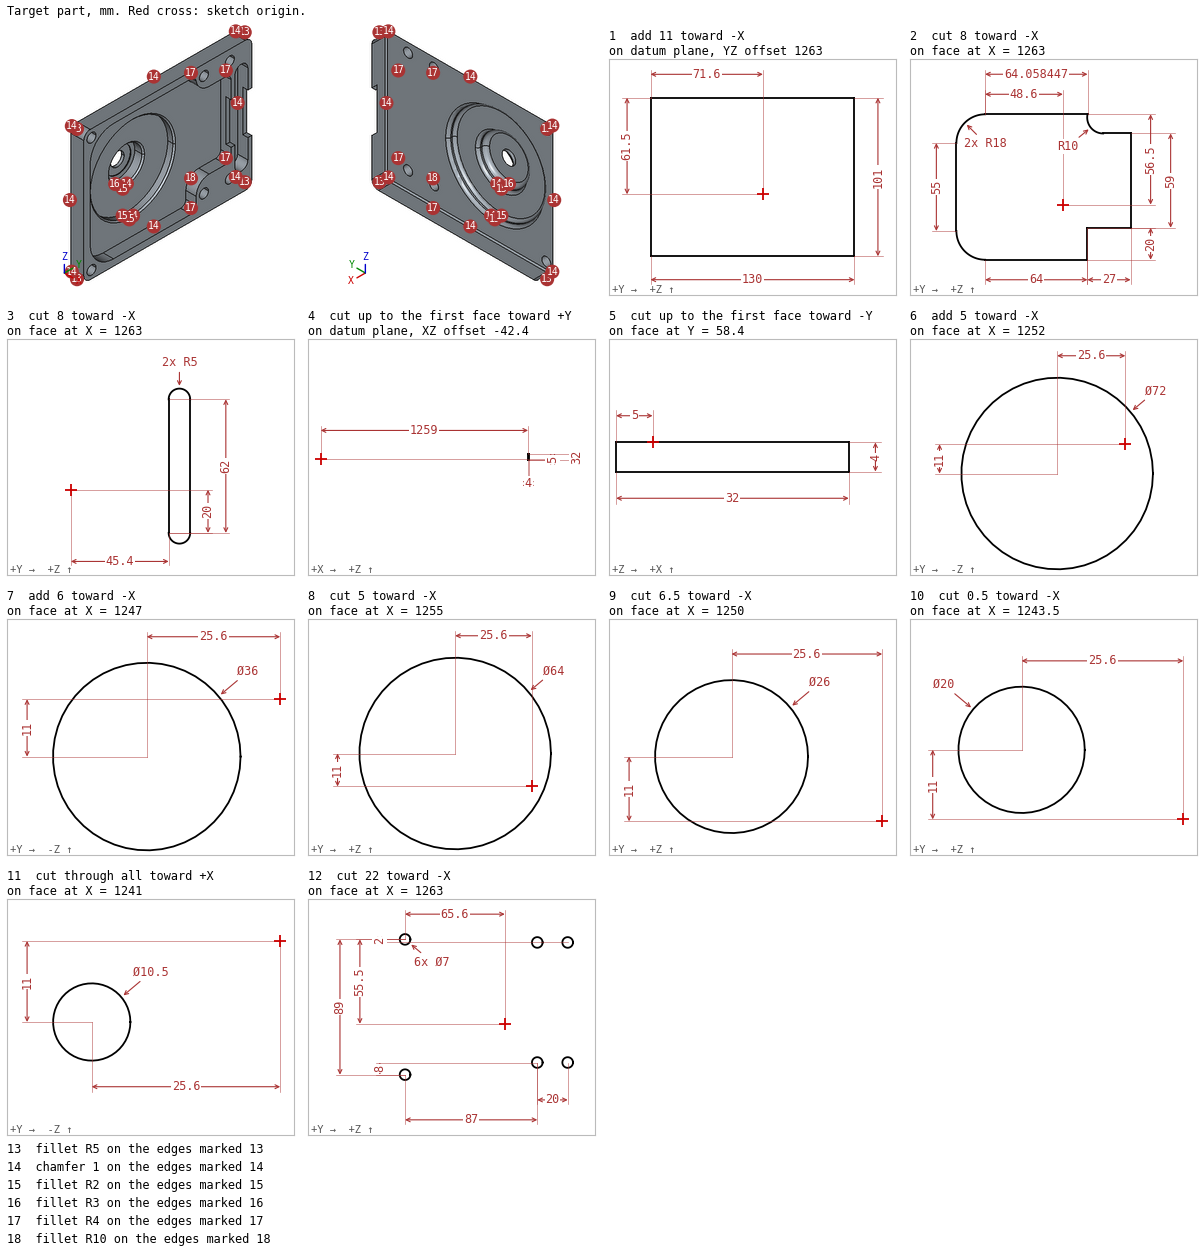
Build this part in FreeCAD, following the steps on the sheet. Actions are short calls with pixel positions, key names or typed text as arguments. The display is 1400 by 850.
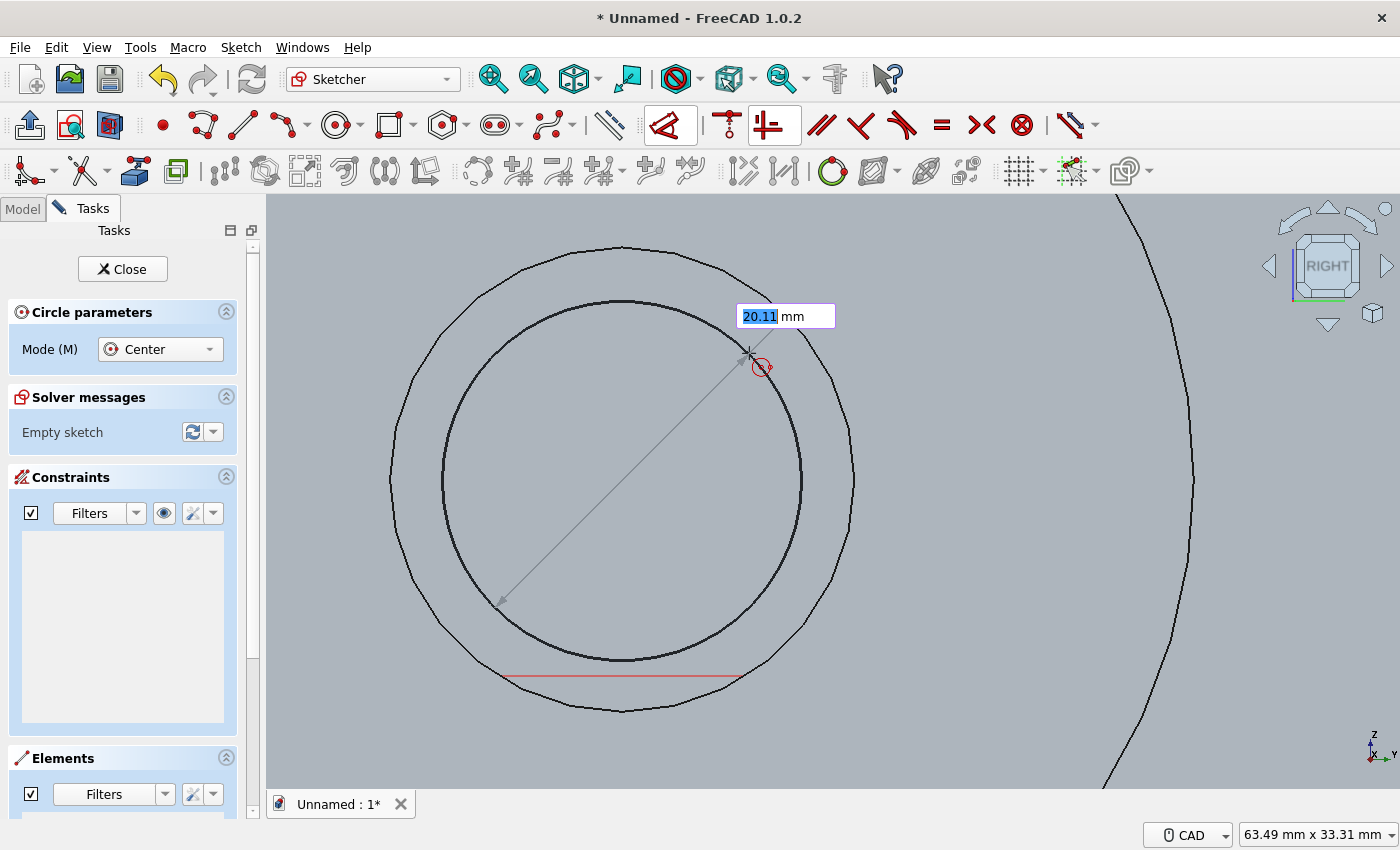
text(20)
key(Return)
key(Escape)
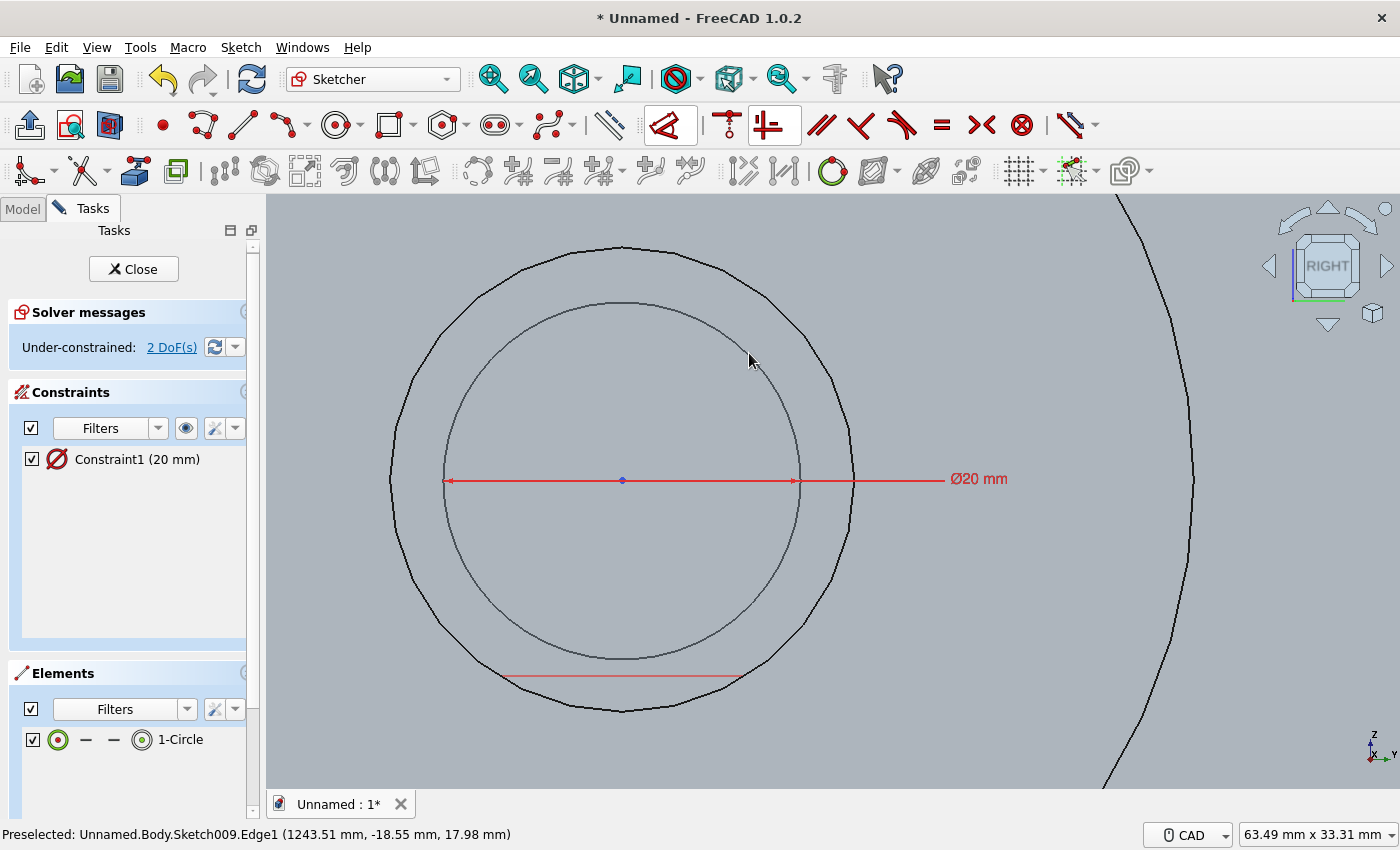
click(622, 481)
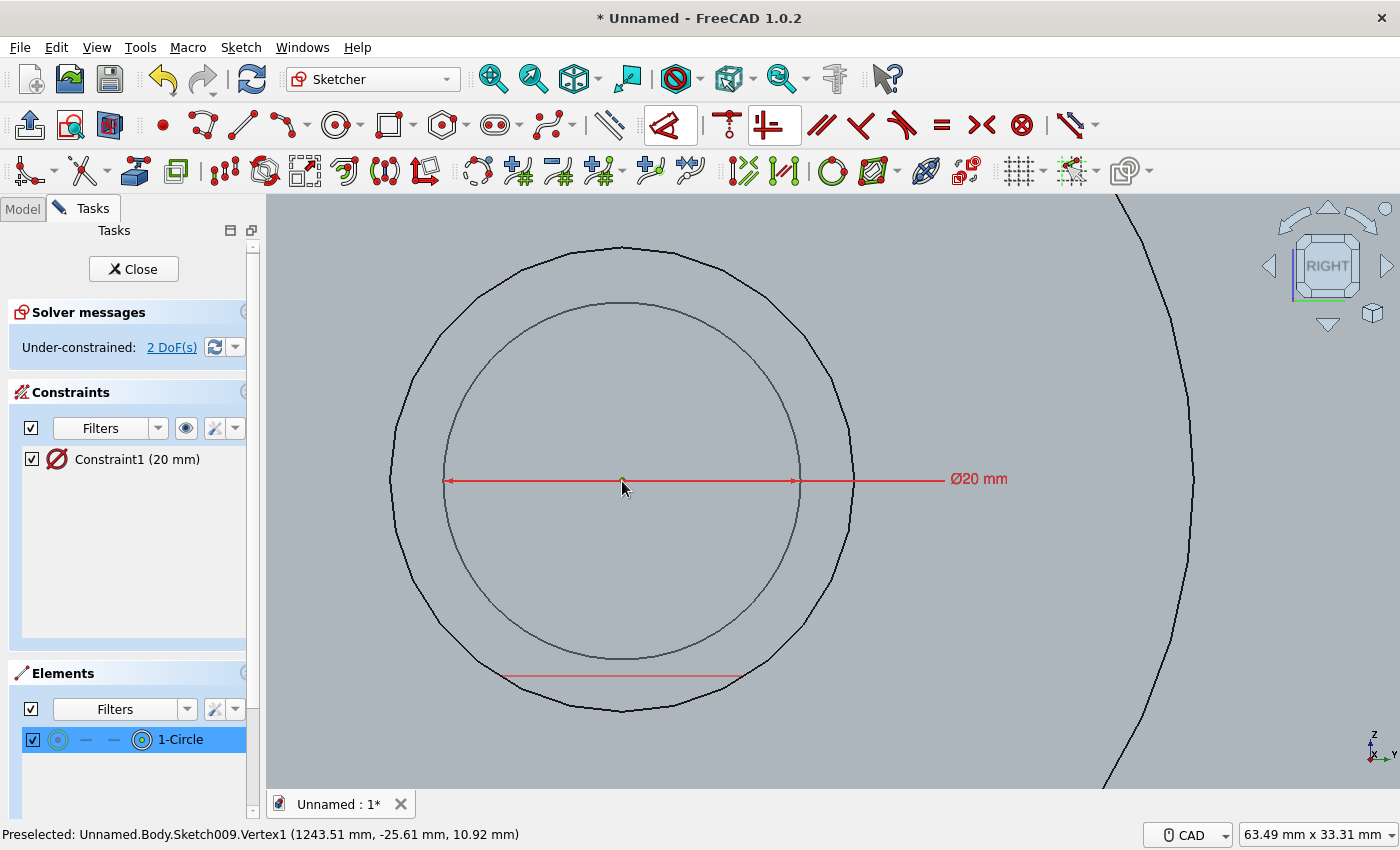
key(i)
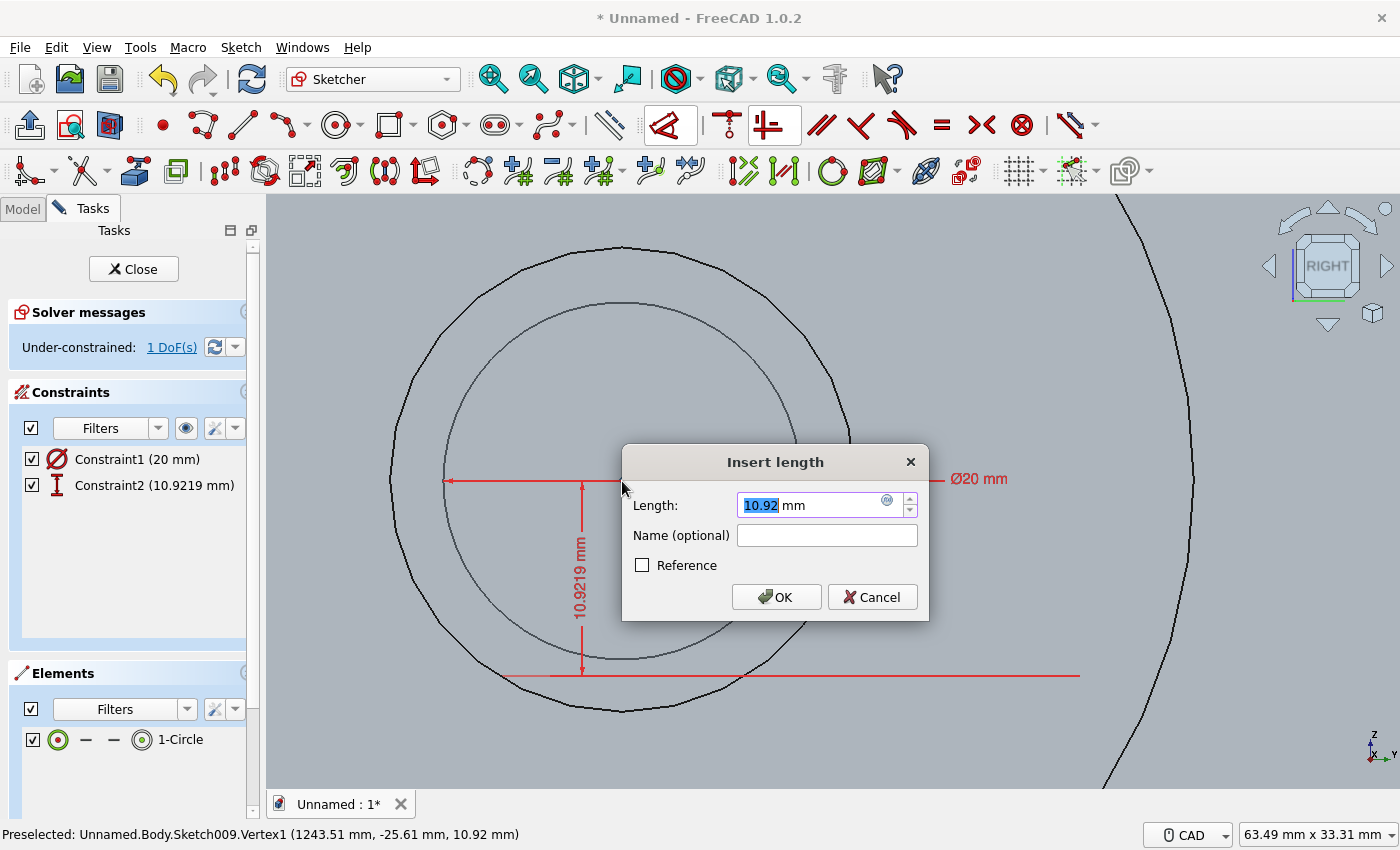
text(11)
key(Return)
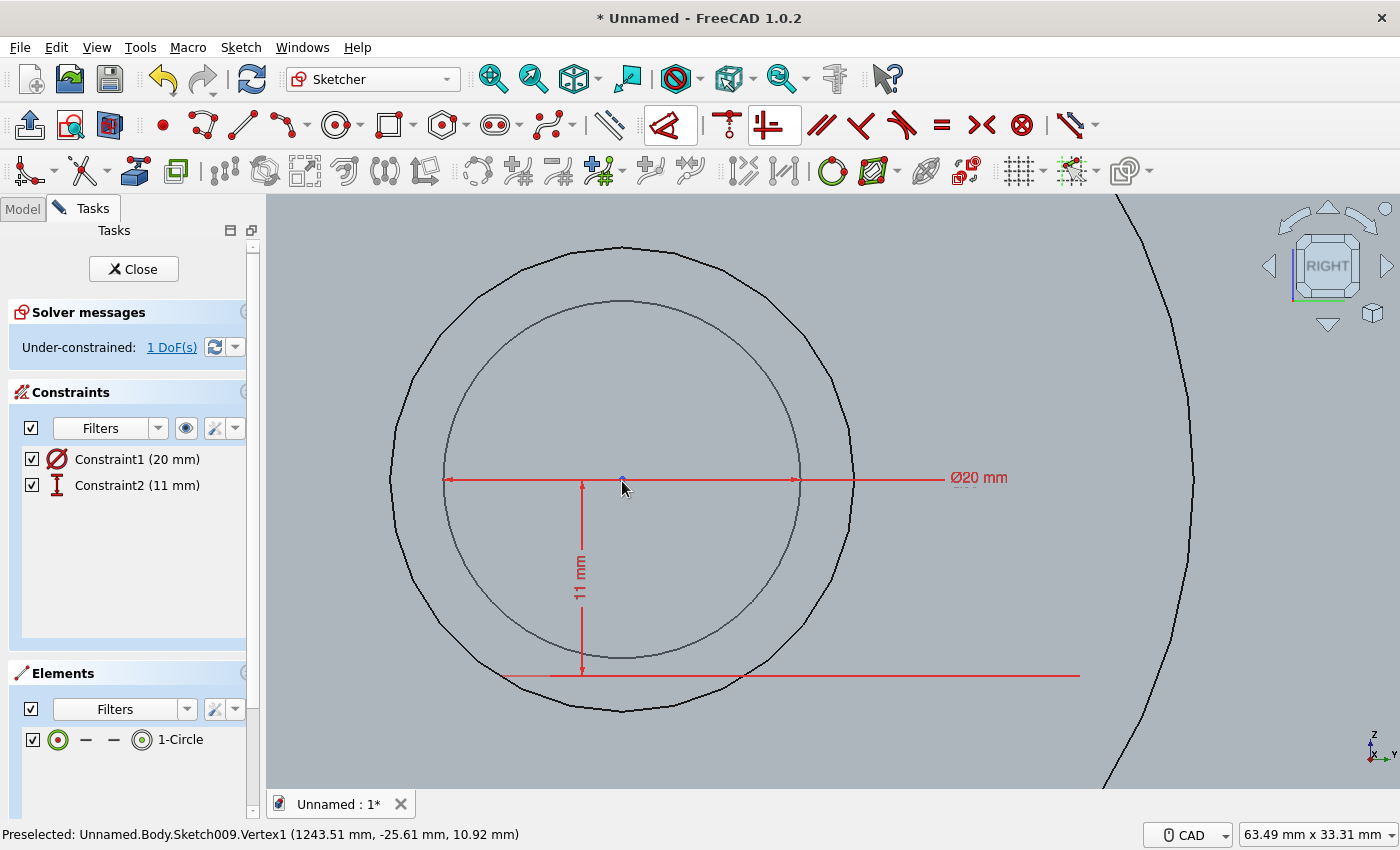
click(622, 480)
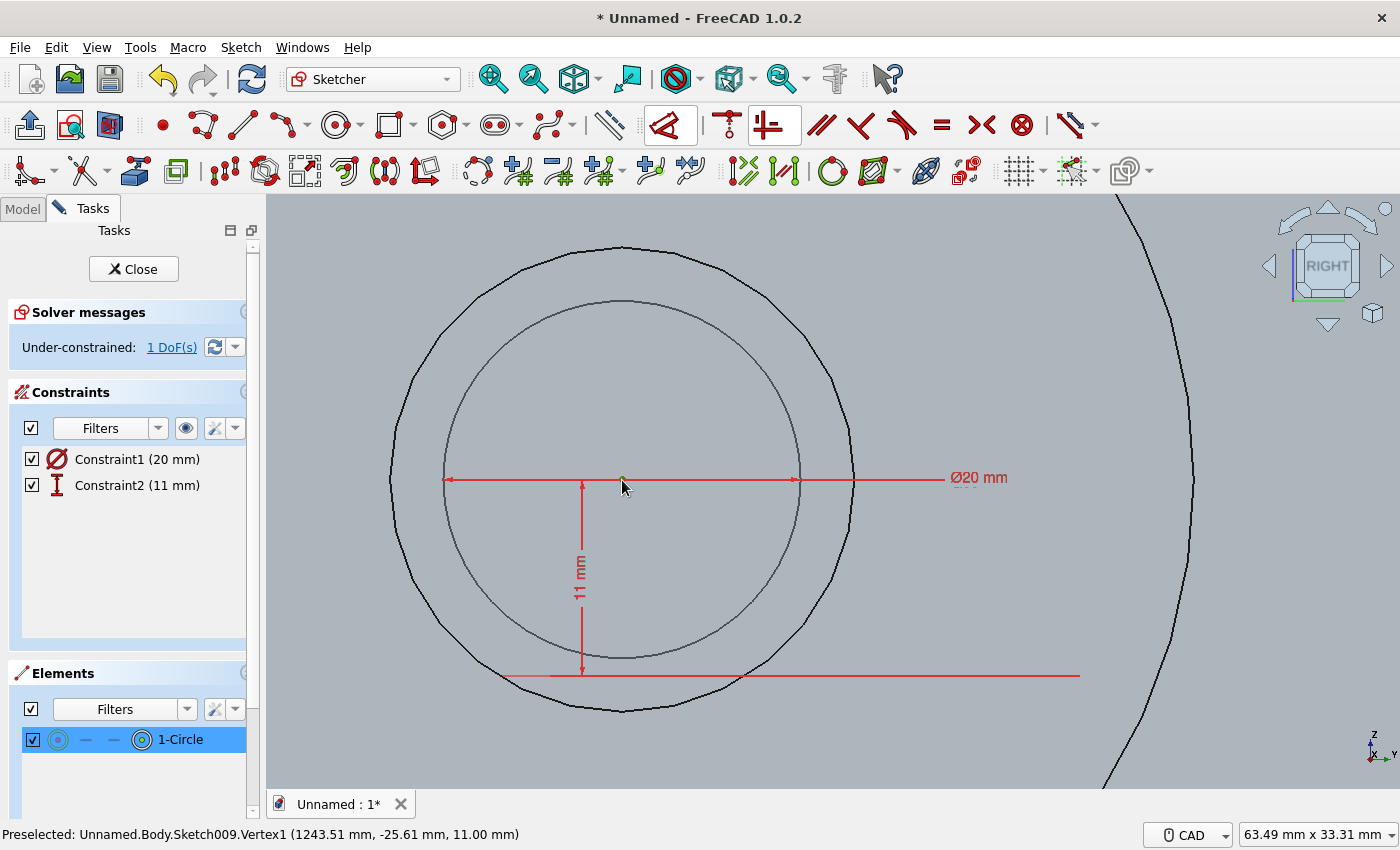
key(l)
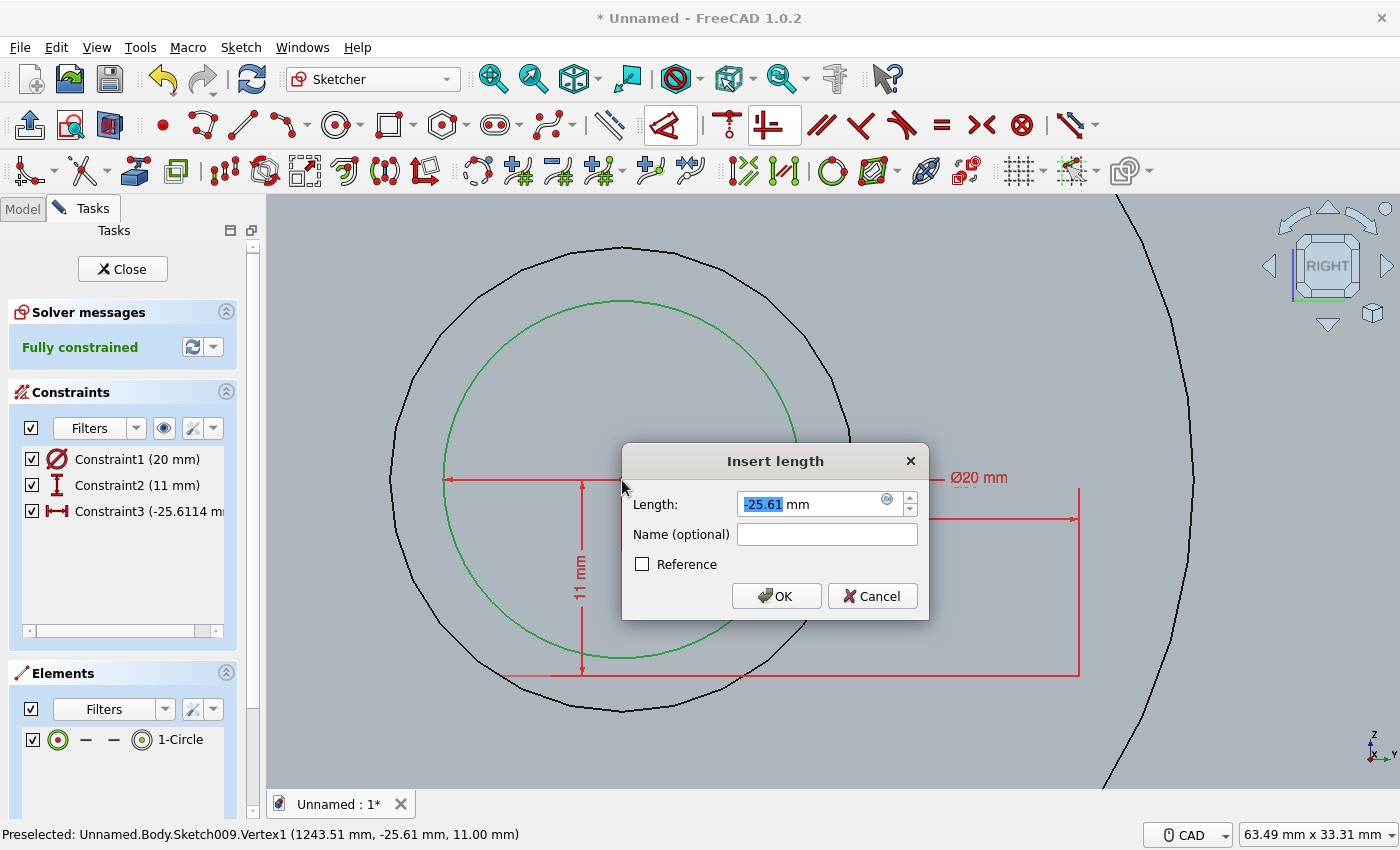
text(-25.6)
key(Return)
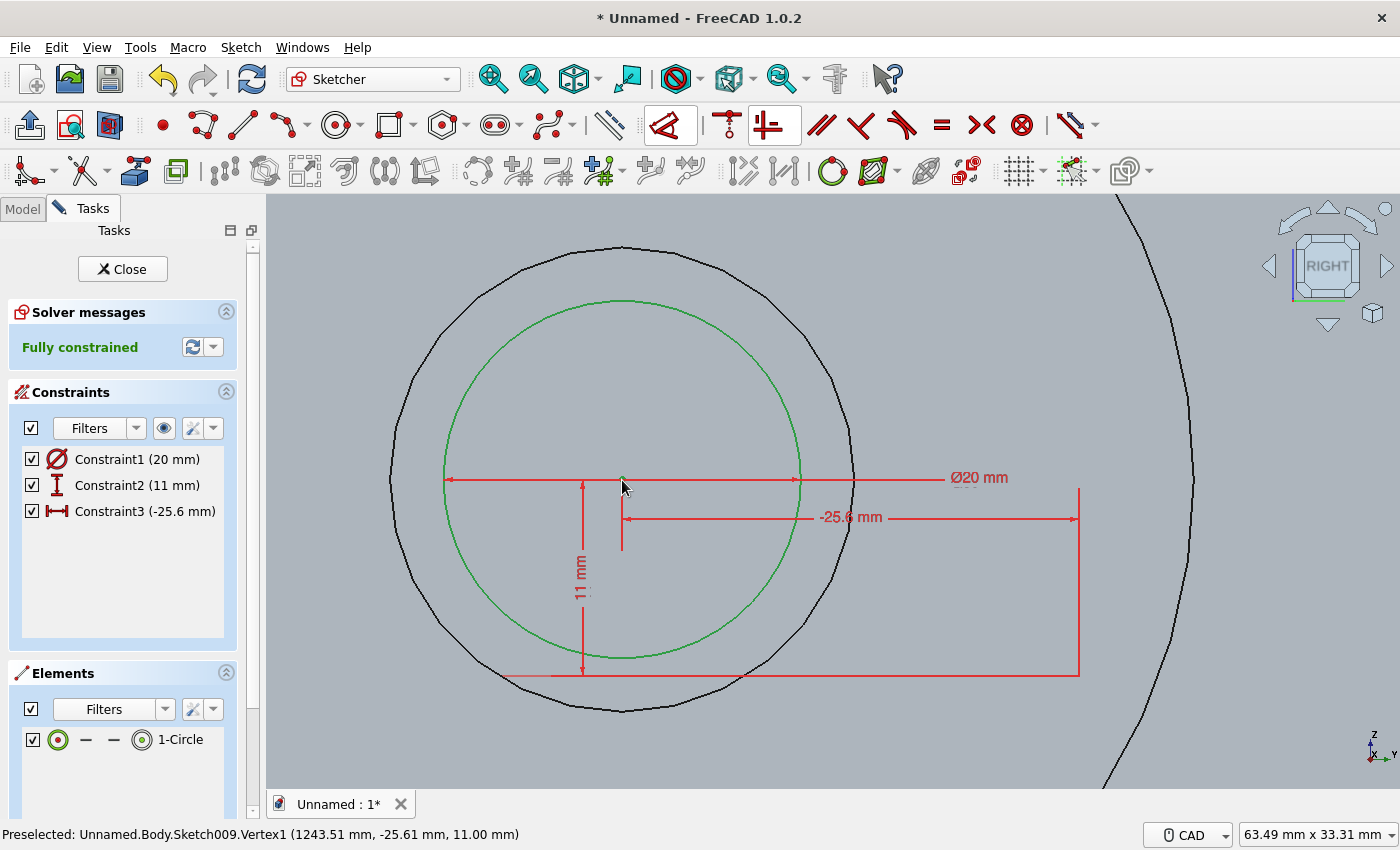
click(123, 269)